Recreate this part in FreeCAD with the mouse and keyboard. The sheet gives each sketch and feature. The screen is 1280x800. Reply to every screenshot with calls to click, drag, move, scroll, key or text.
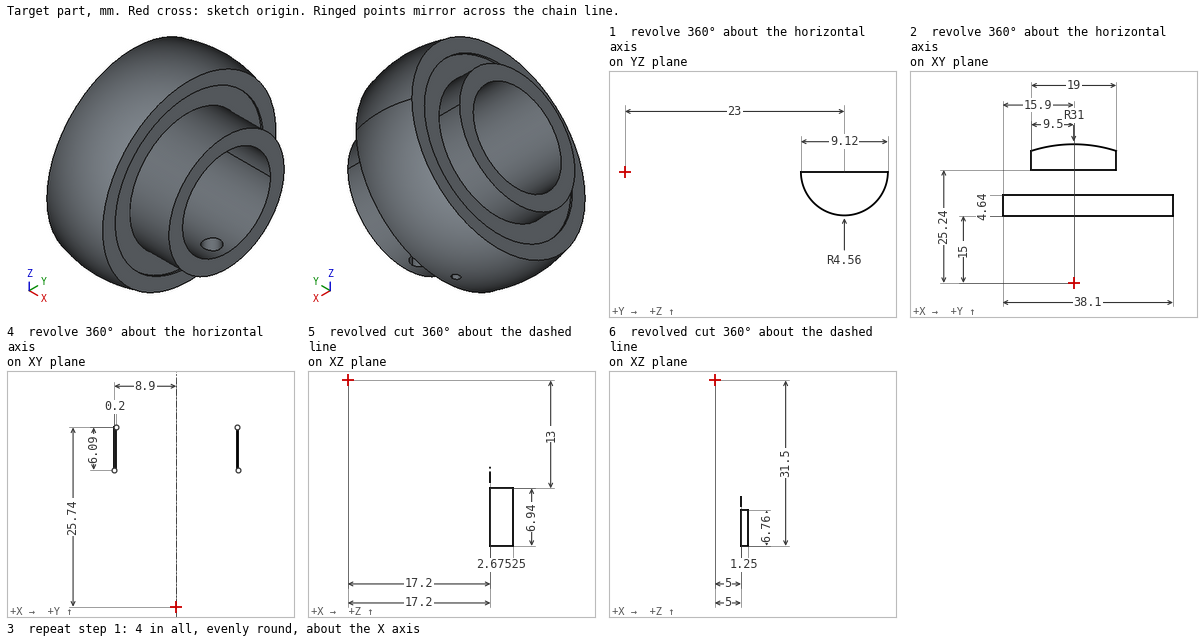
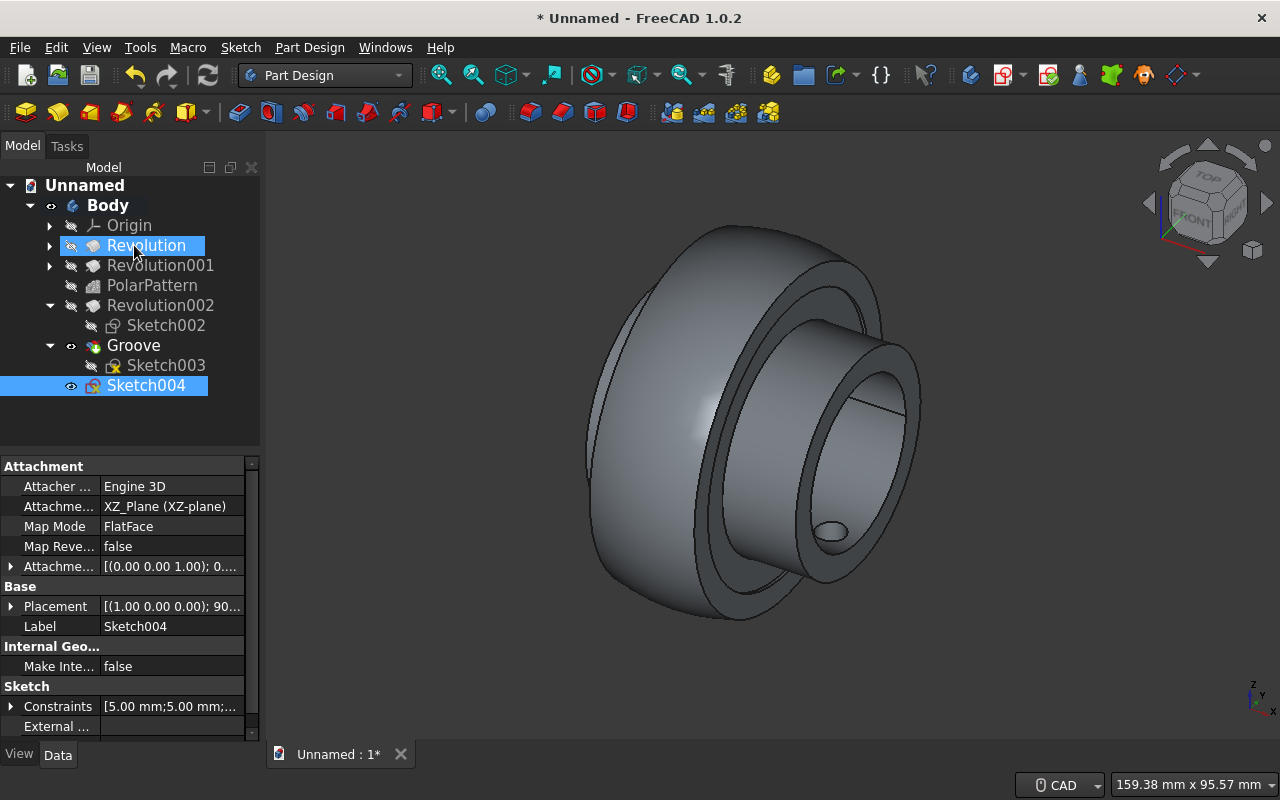
click(304, 112)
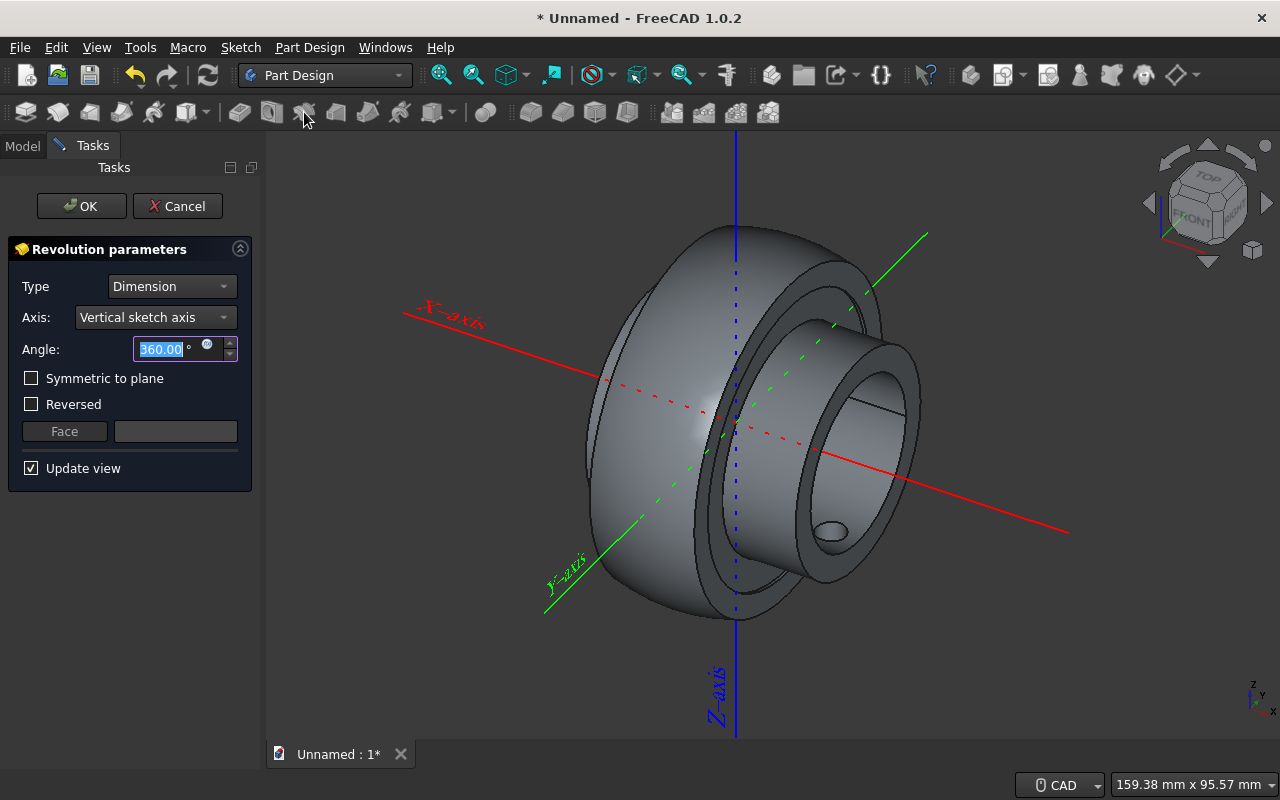
click(156, 318)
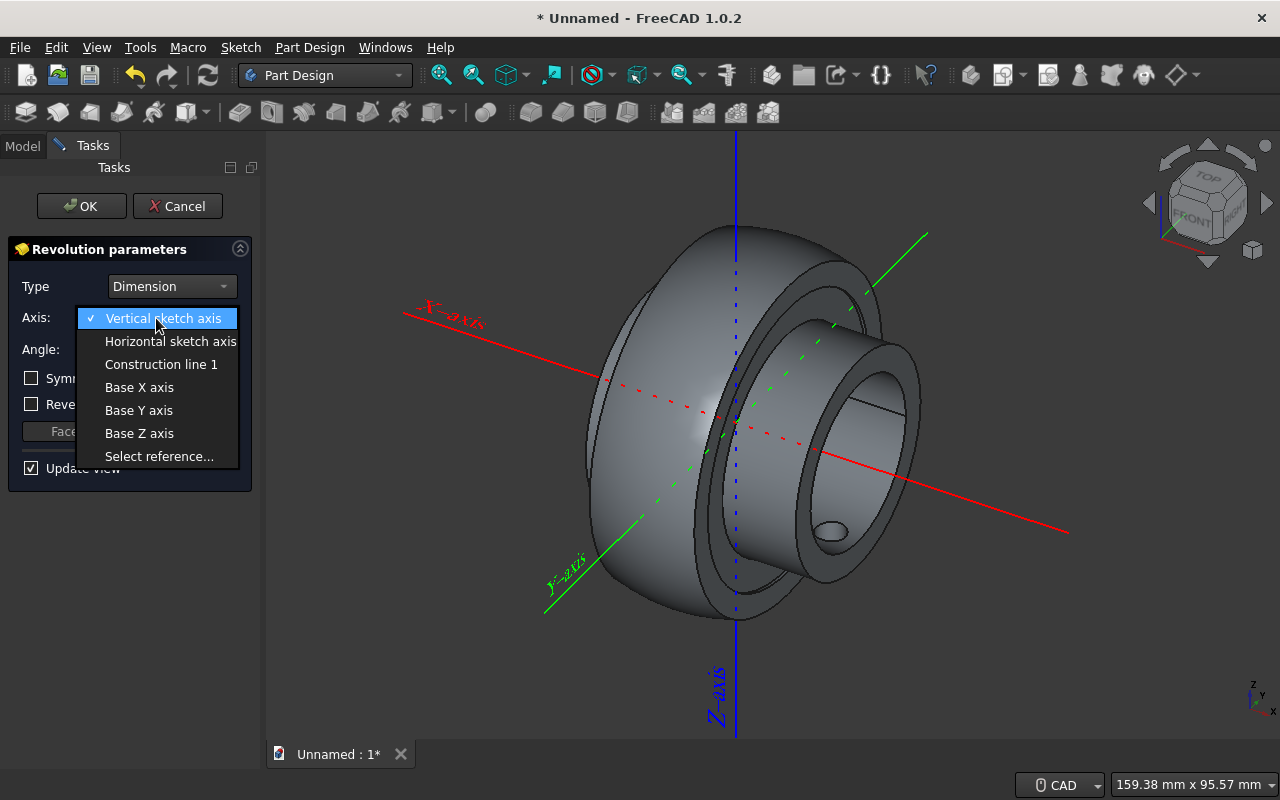
click(156, 364)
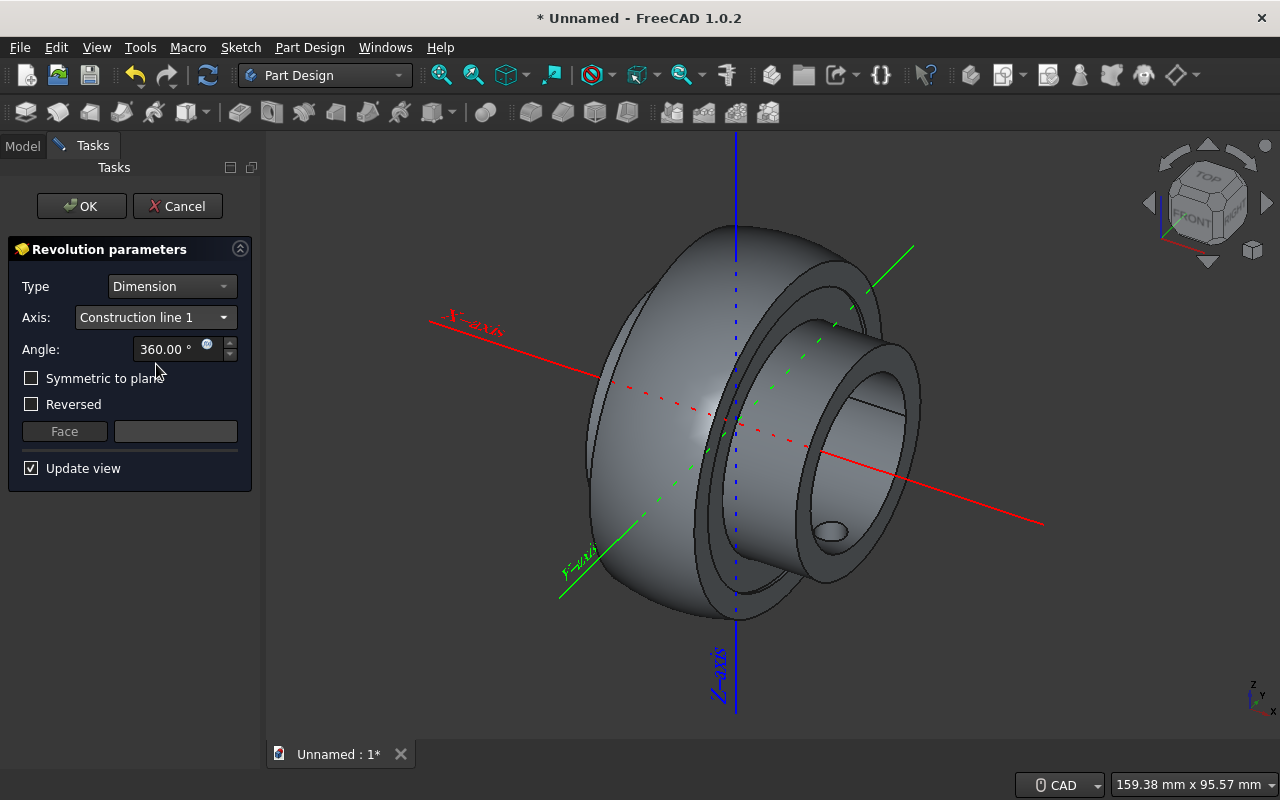
click(82, 206)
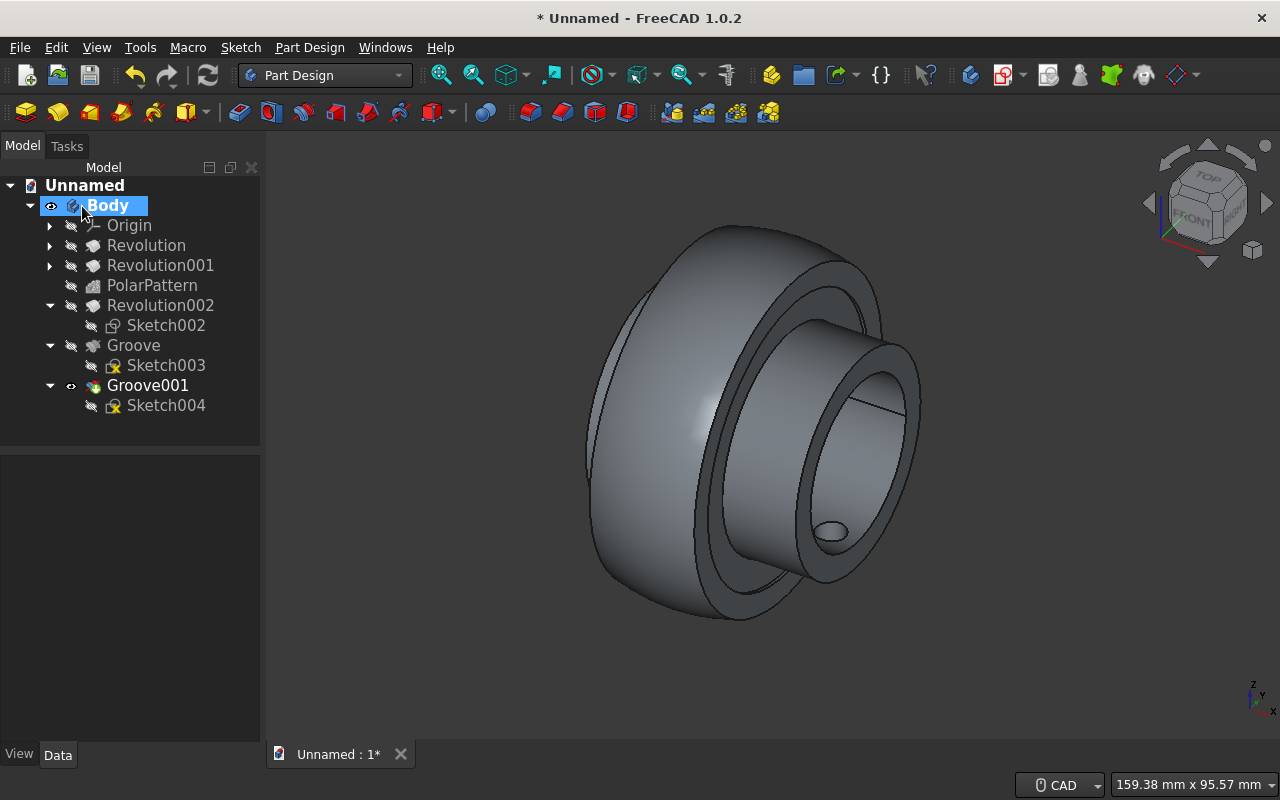
key(0)